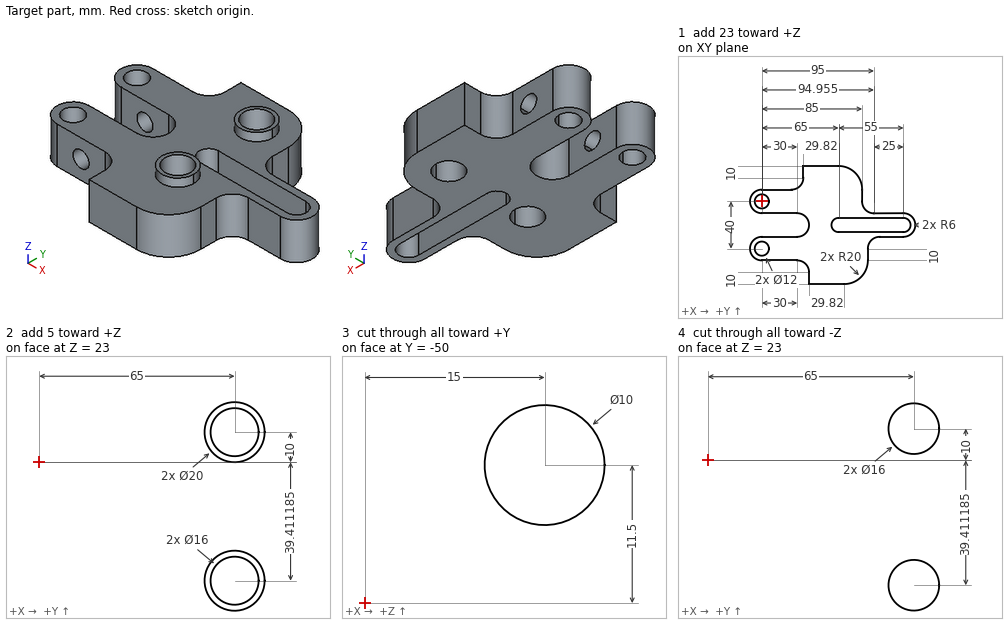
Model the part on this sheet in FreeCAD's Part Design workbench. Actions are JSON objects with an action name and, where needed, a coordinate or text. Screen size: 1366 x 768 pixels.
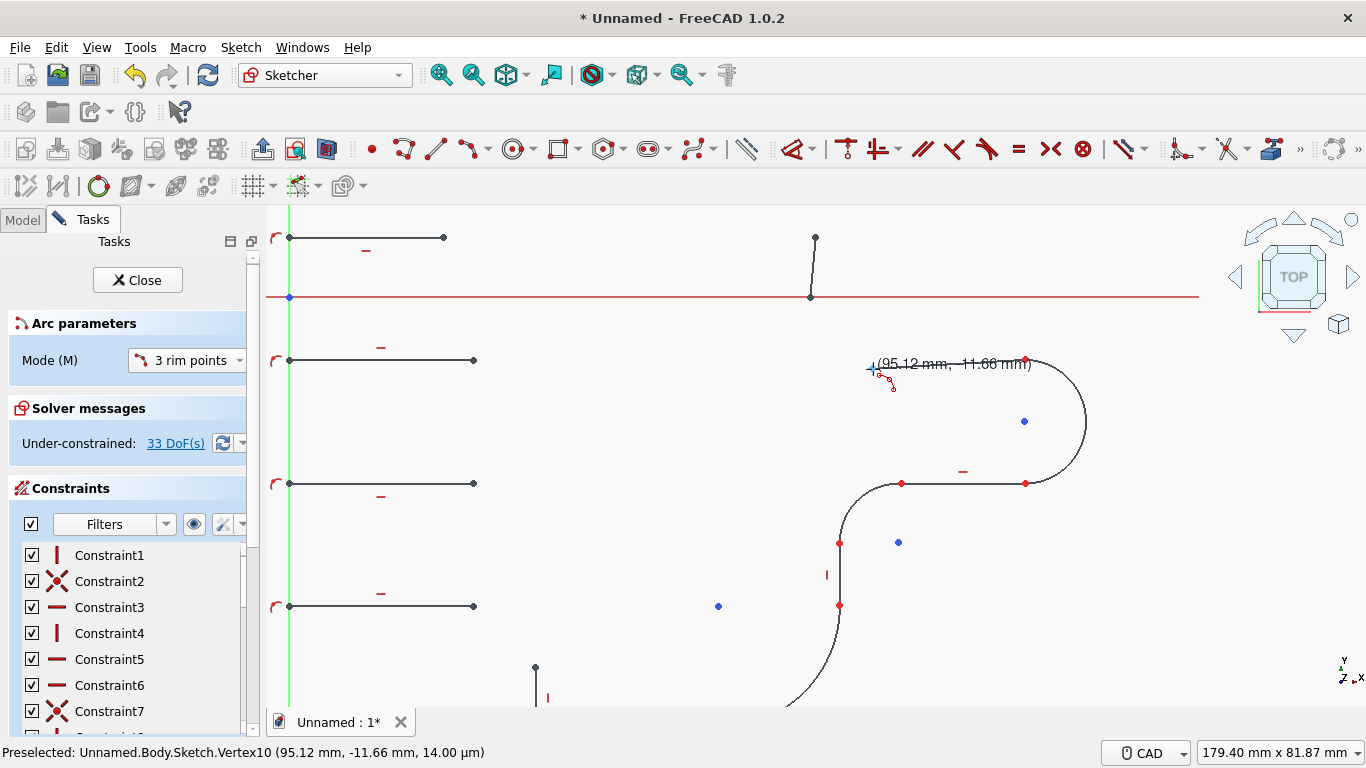
{"action": "scroll", "coordinate": [810, 298], "scroll_direction": "up", "scroll_amount": 19}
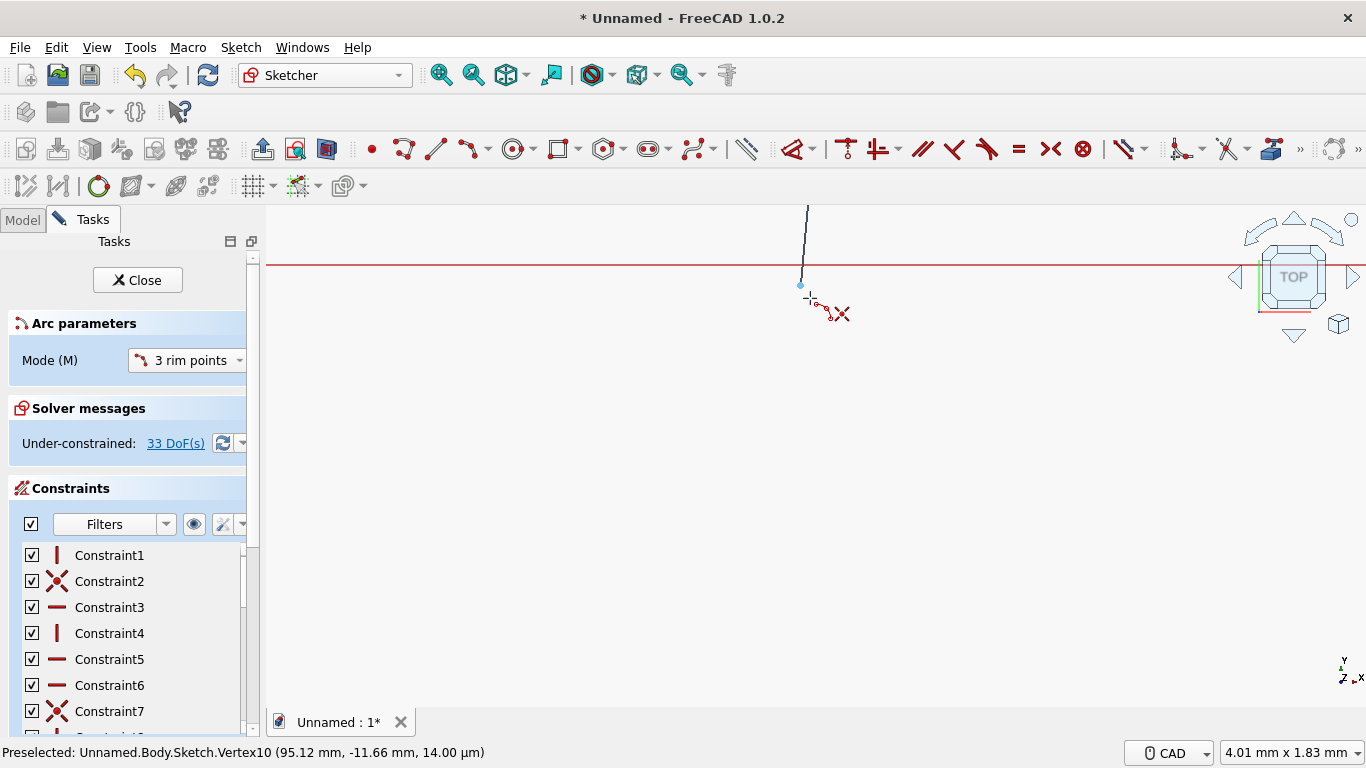
{"action": "left_click", "coordinate": [801, 285]}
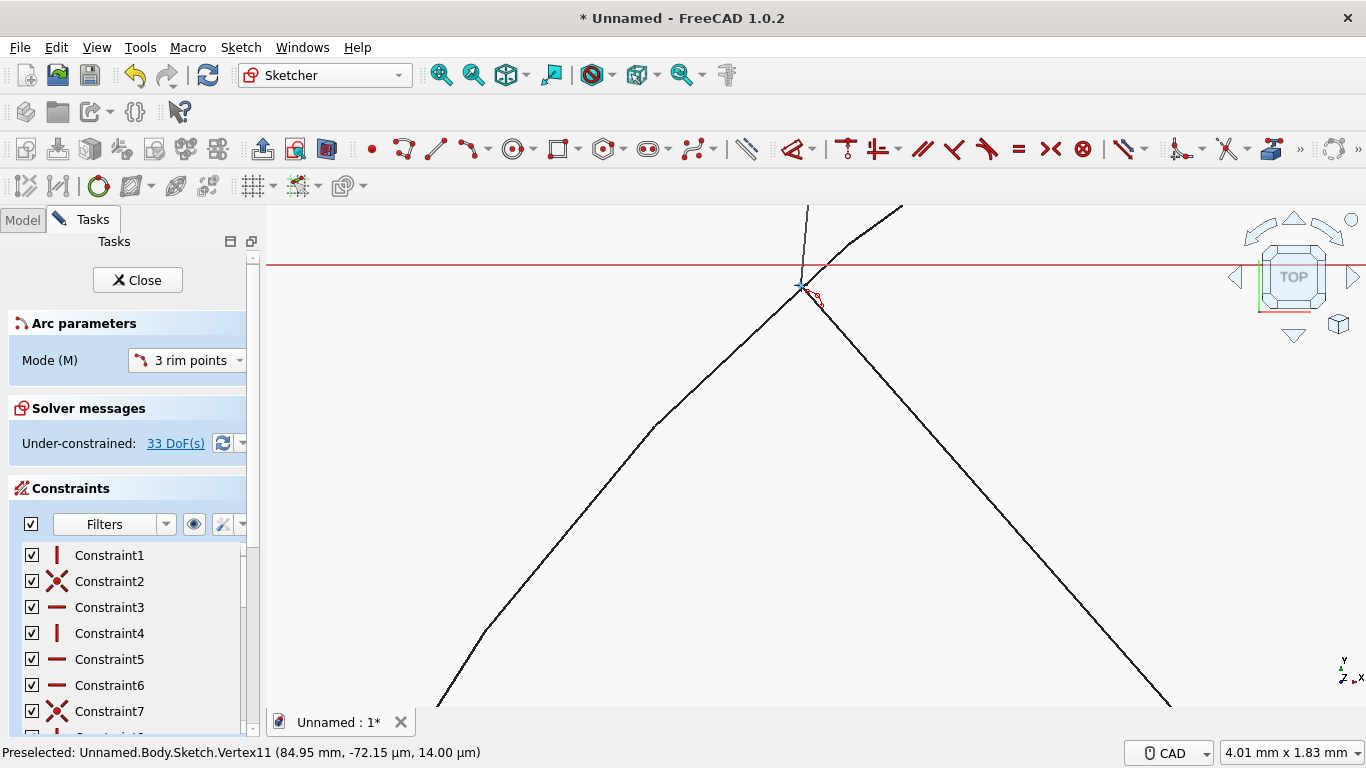
{"action": "scroll", "coordinate": [748, 456], "scroll_direction": "down", "scroll_amount": 15}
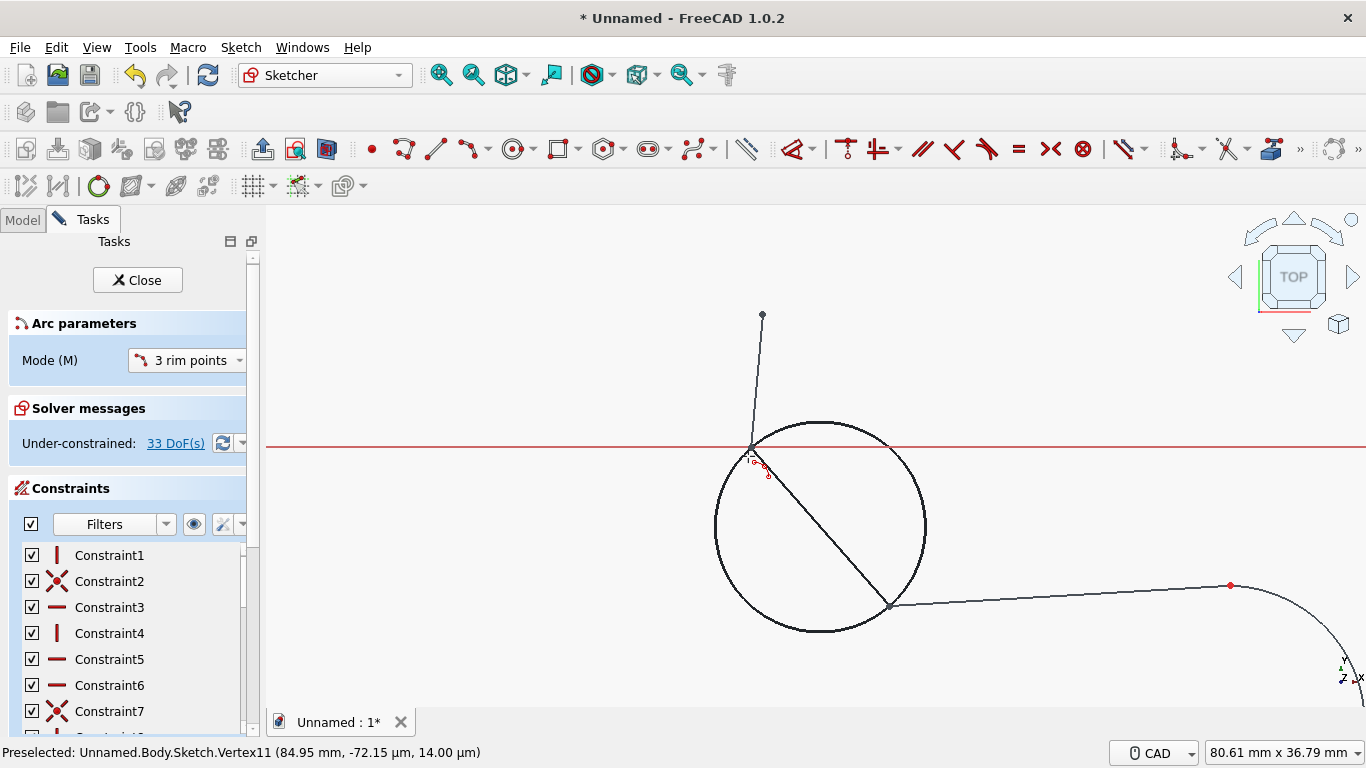
{"action": "scroll", "coordinate": [858, 370], "scroll_direction": "down", "scroll_amount": 7}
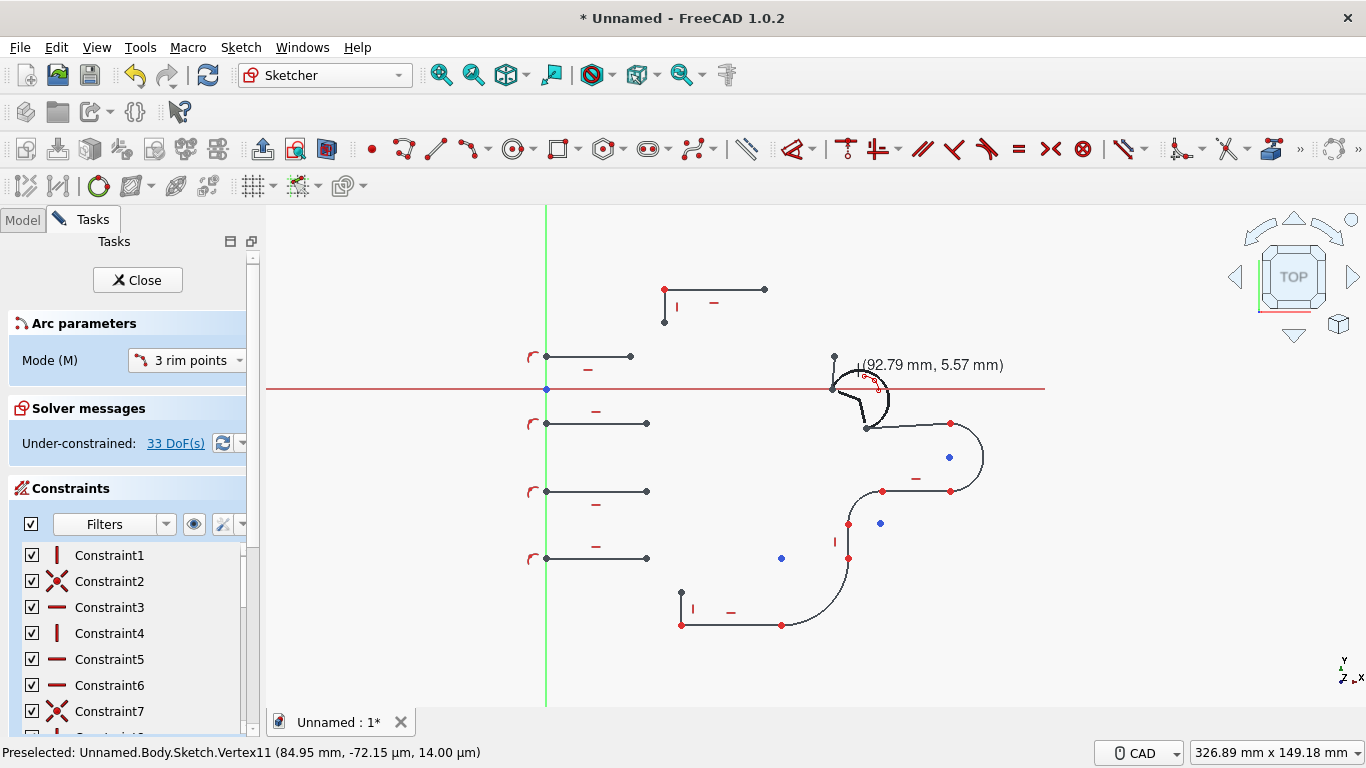
{"action": "scroll", "coordinate": [842, 413], "scroll_direction": "up", "scroll_amount": 3}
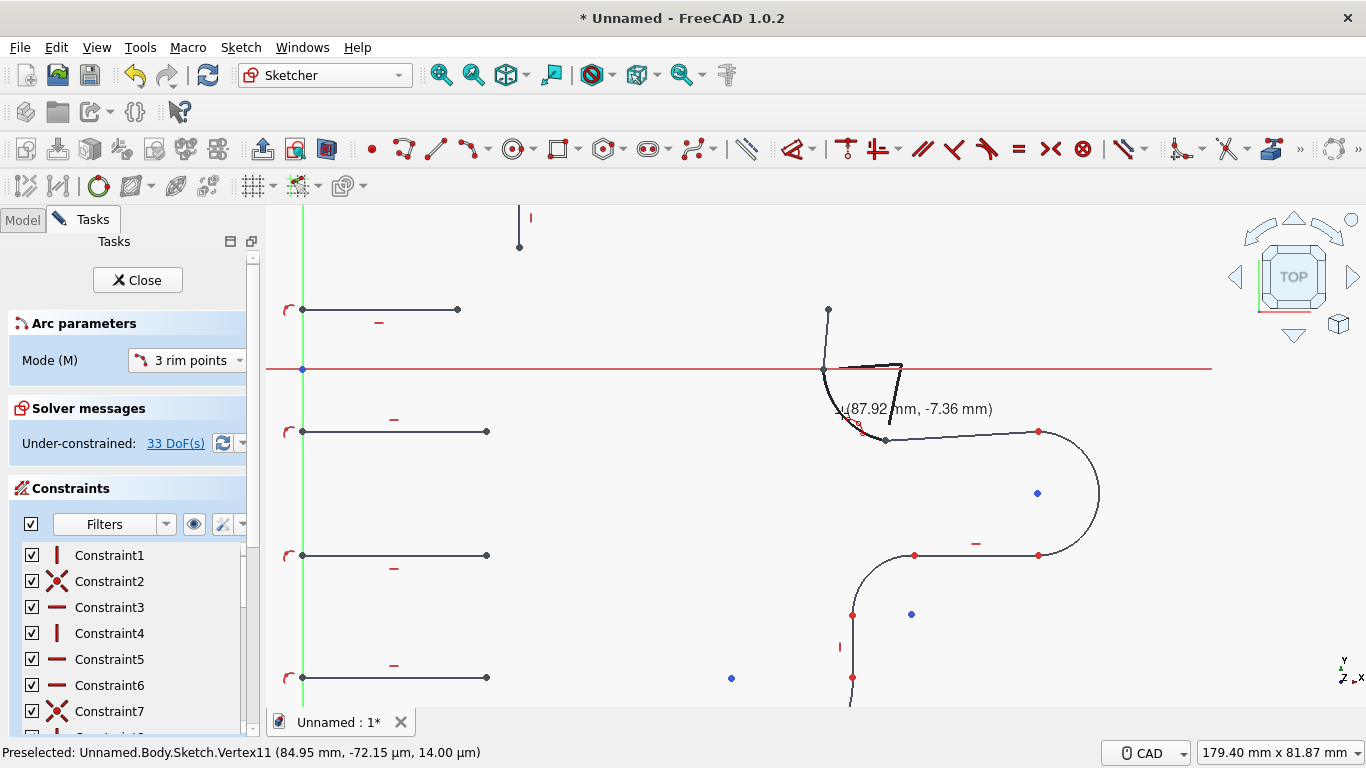
{"action": "left_click", "coordinate": [841, 413]}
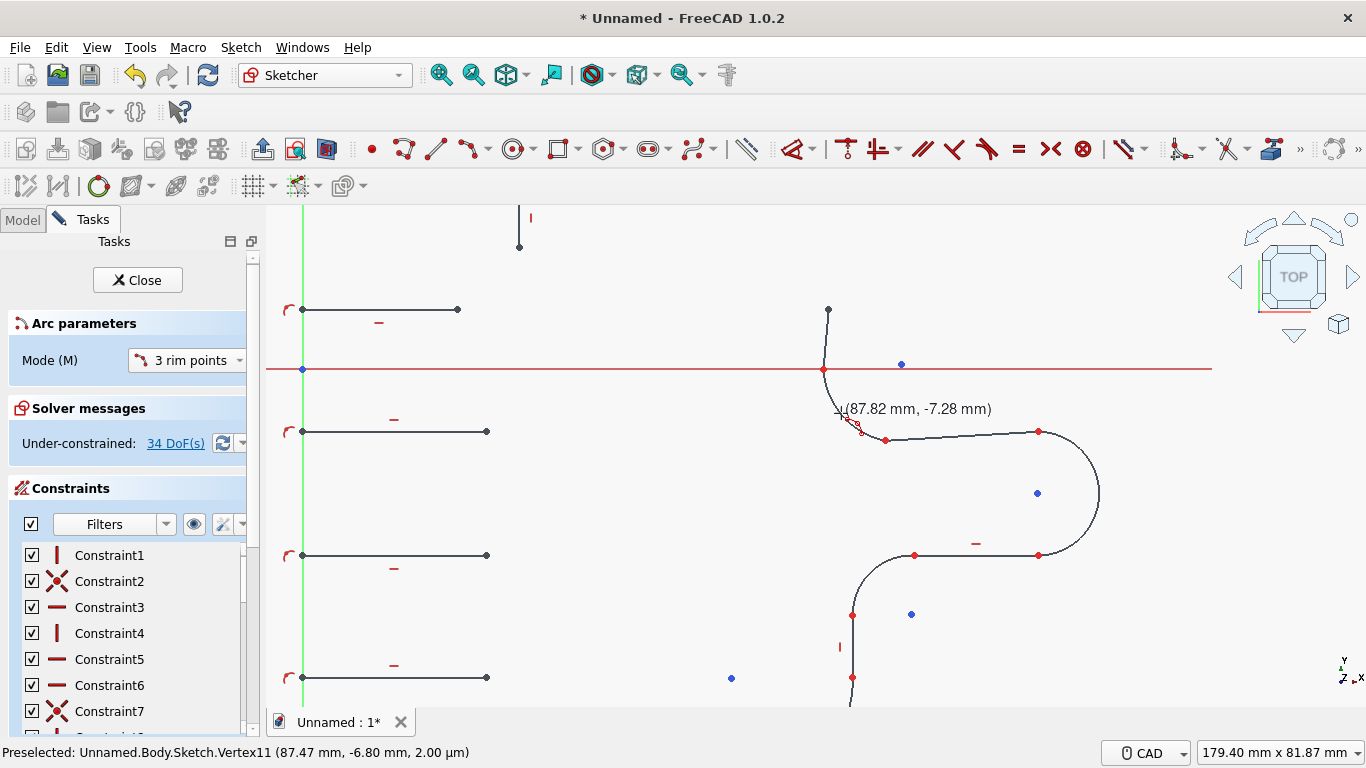
{"action": "left_click", "coordinate": [829, 310]}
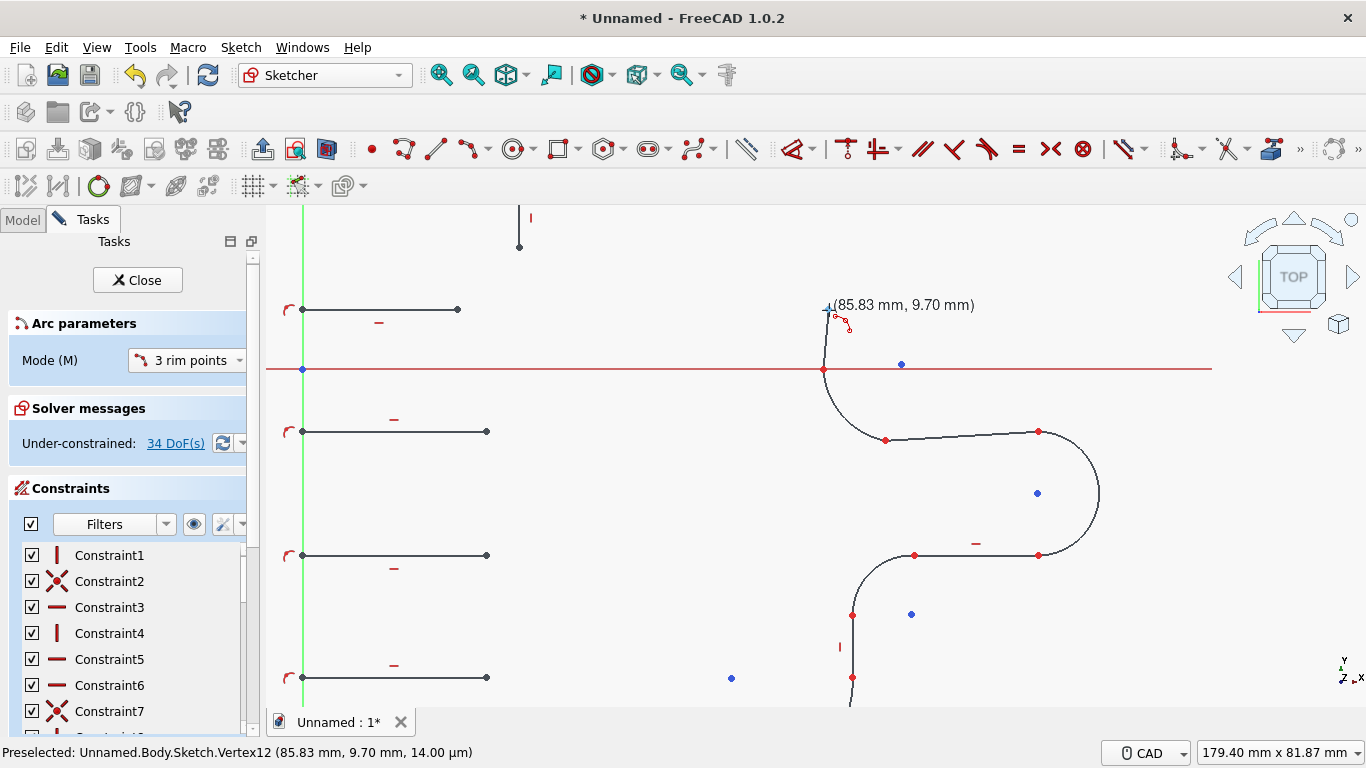
{"action": "scroll", "coordinate": [841, 412], "scroll_direction": "down", "scroll_amount": 3}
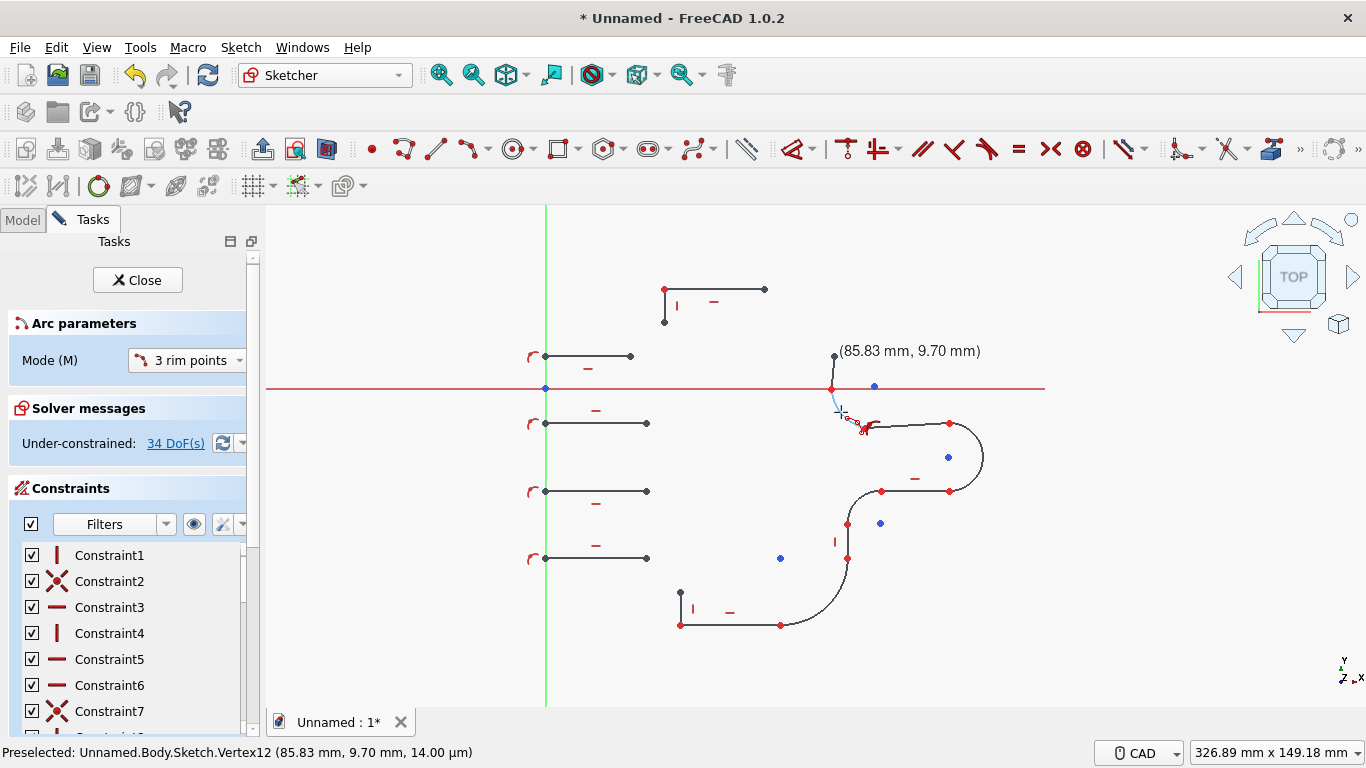
{"action": "left_click", "coordinate": [765, 289]}
{"action": "left_click", "coordinate": [812, 308]}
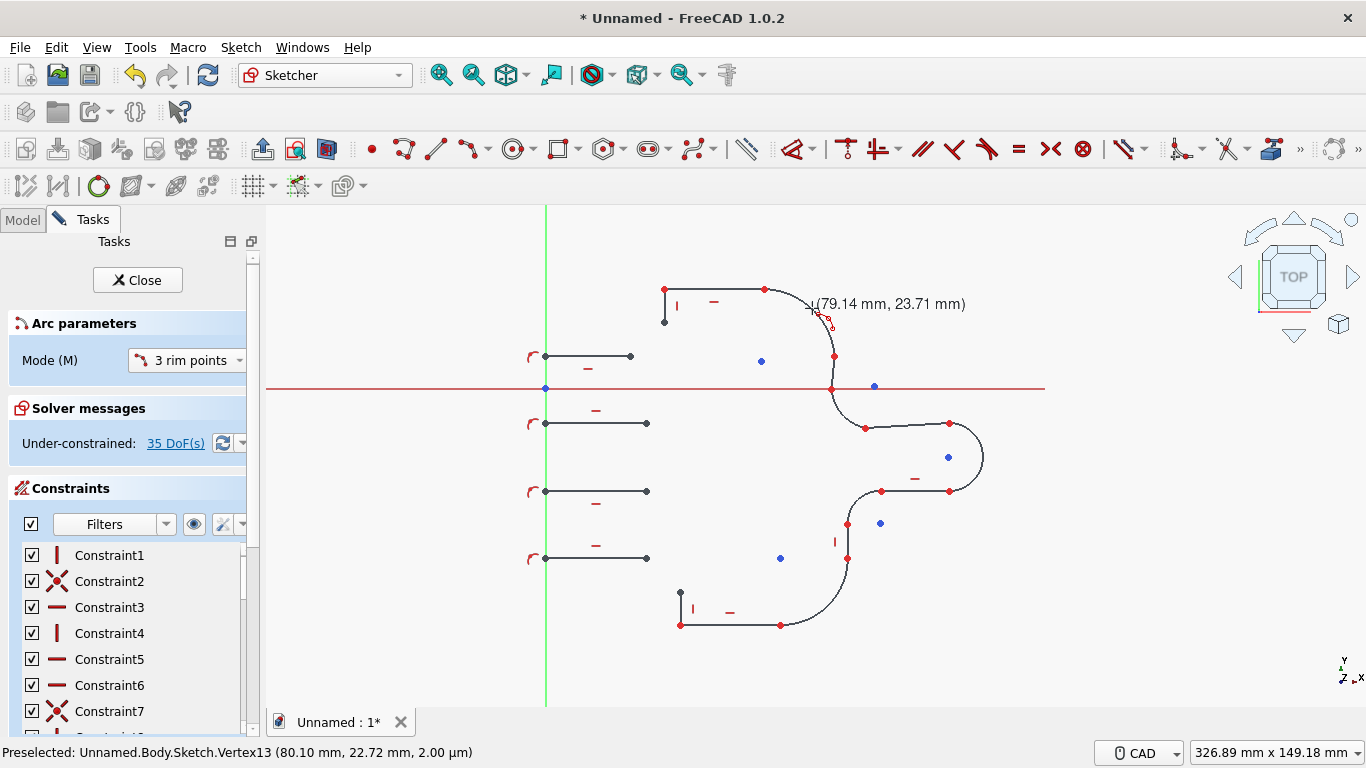
{"action": "left_click", "coordinate": [665, 322]}
{"action": "left_click", "coordinate": [631, 356]}